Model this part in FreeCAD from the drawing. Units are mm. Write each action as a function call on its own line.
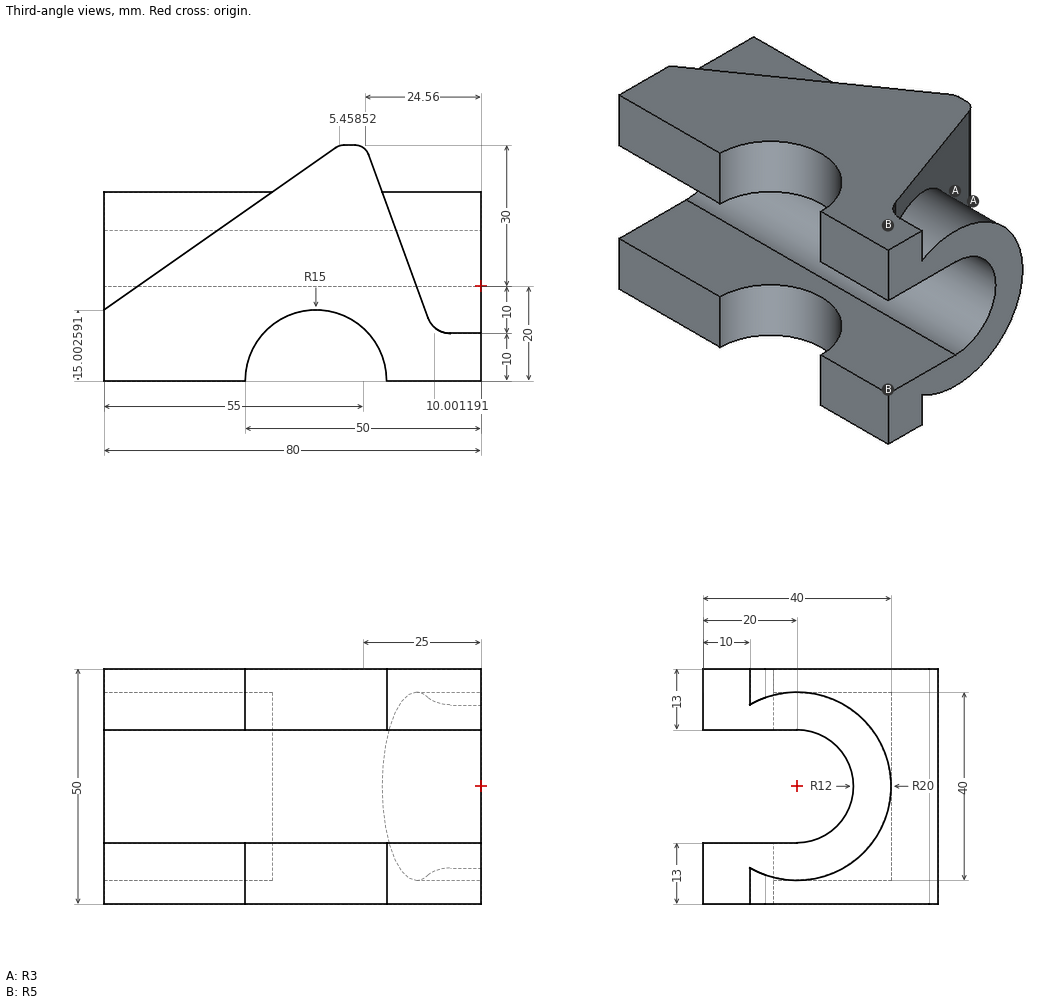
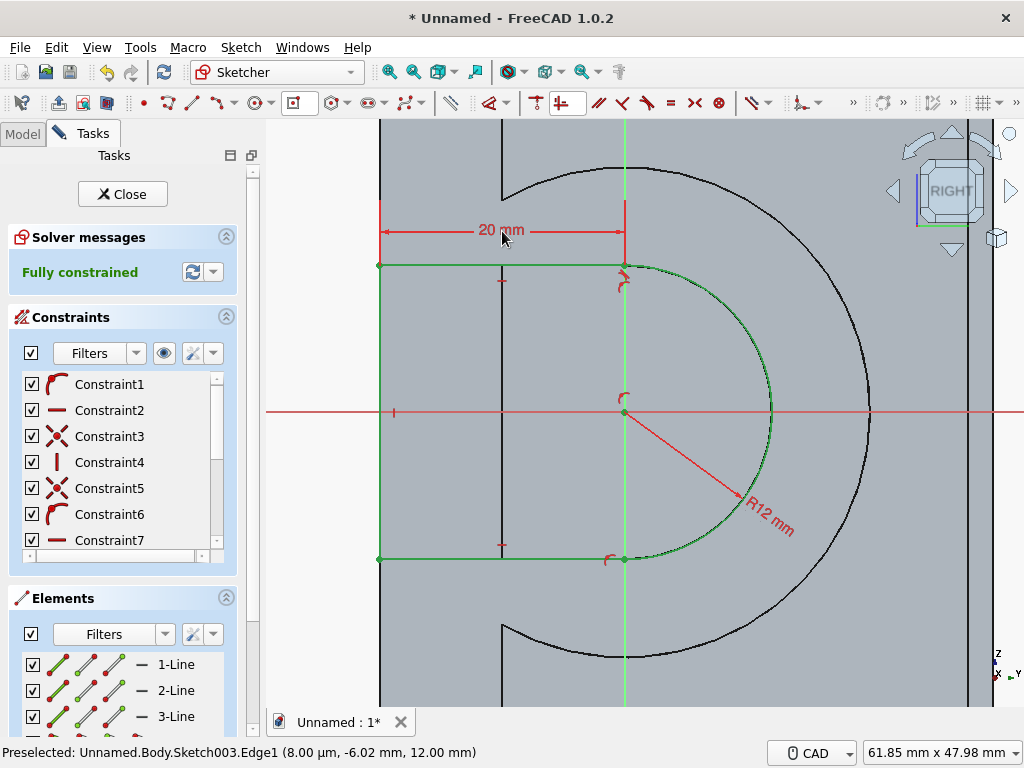
click(123, 194)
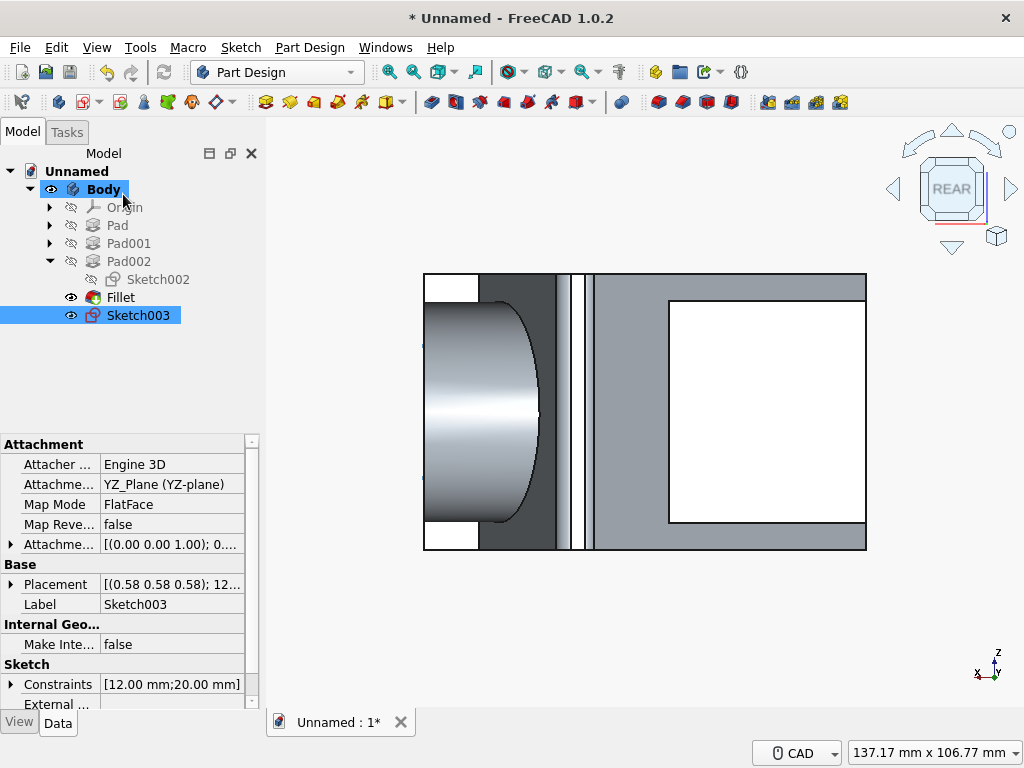
click(432, 102)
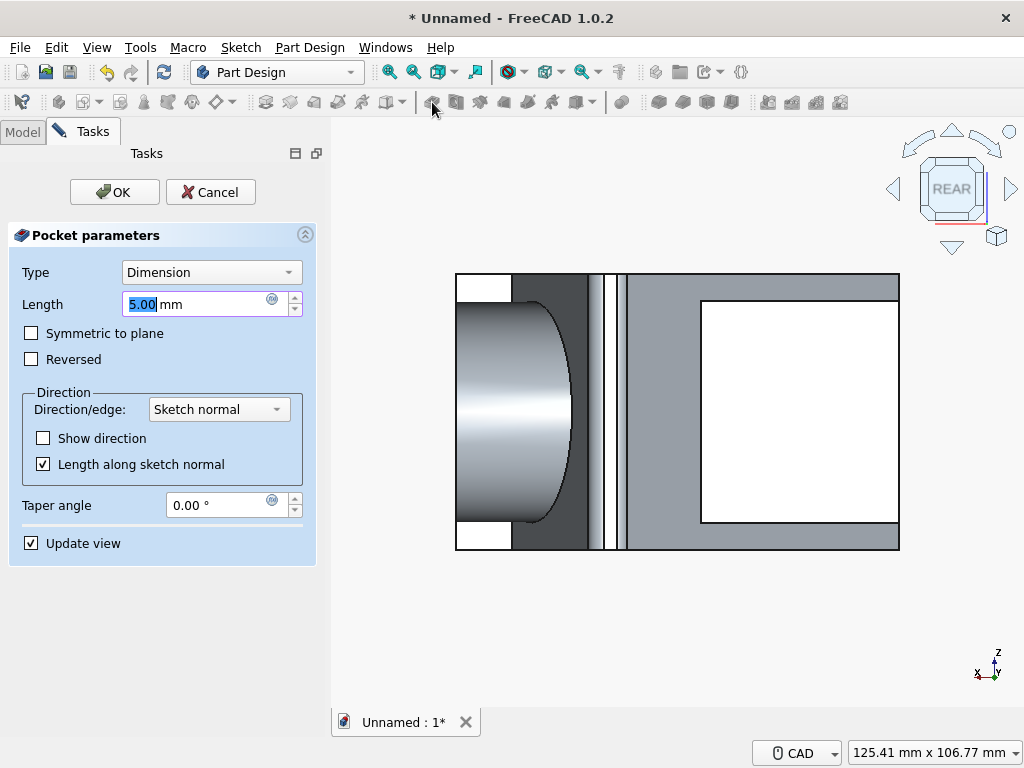
click(212, 272)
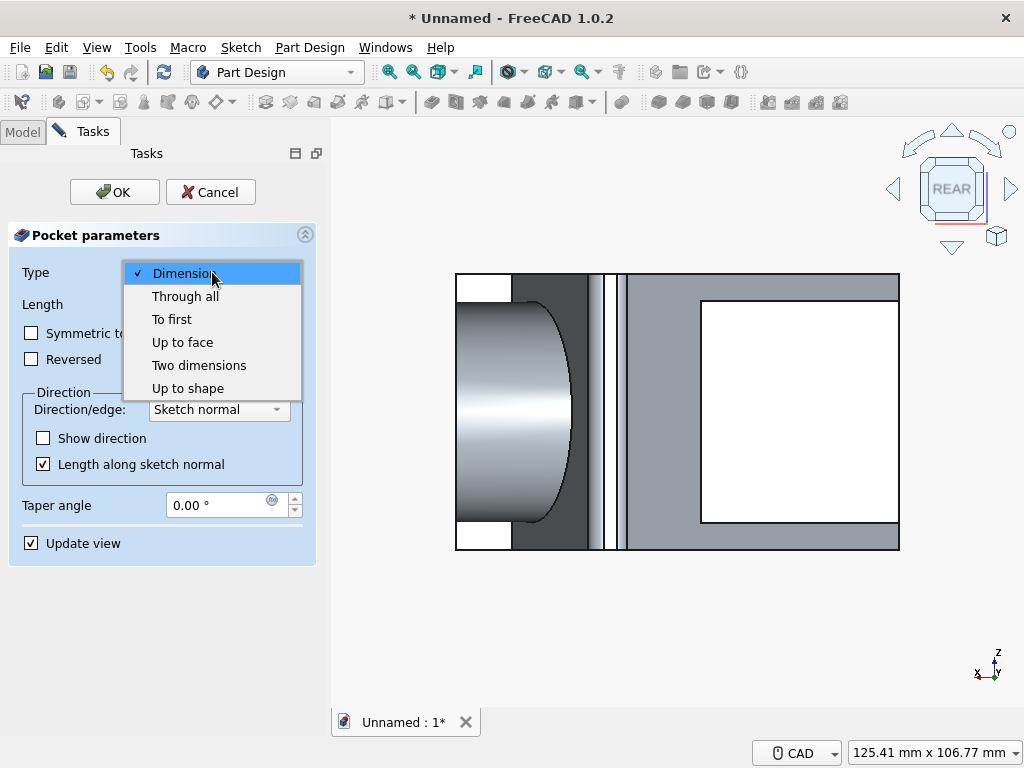
click(212, 296)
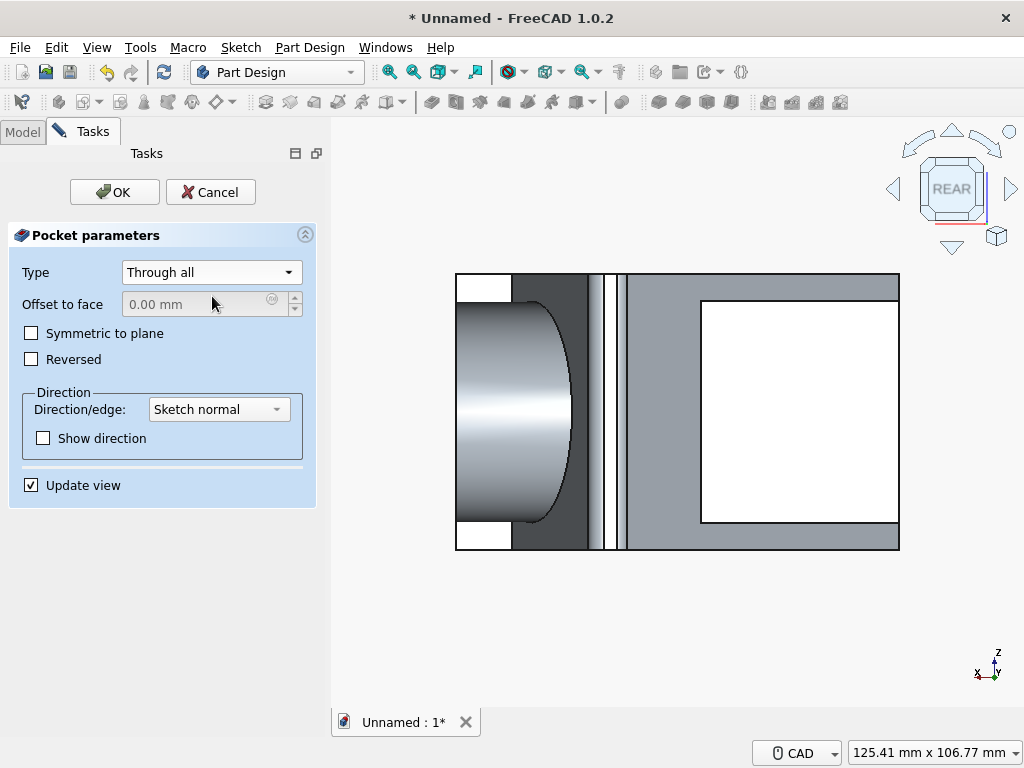
click(115, 192)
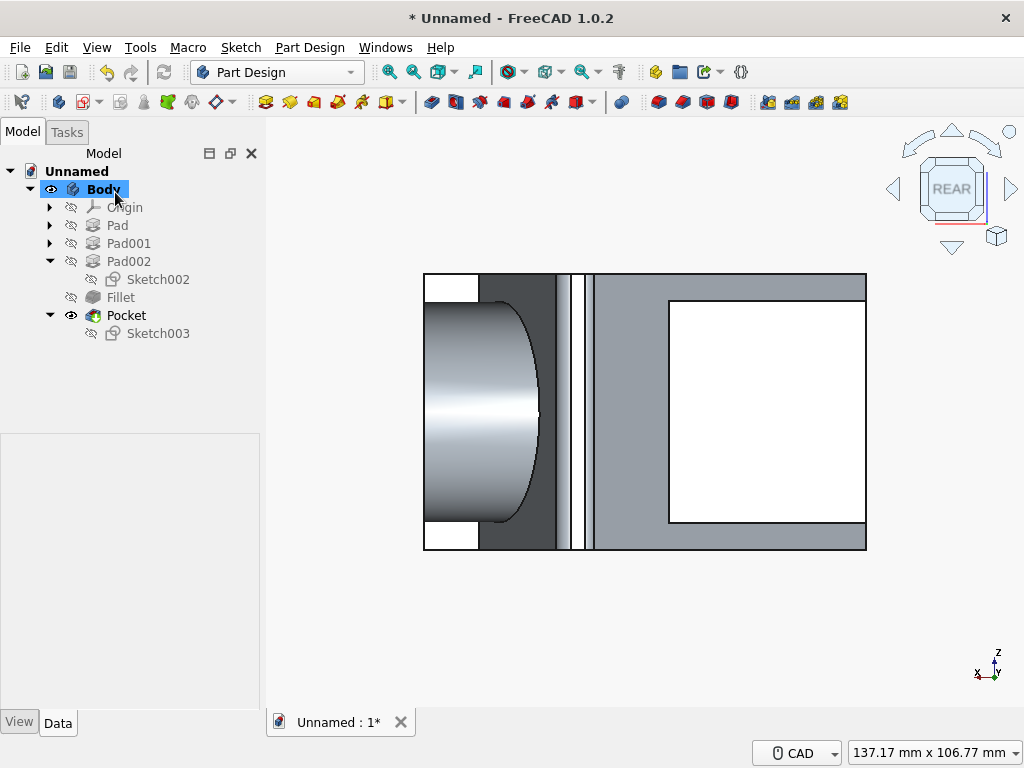
key(0)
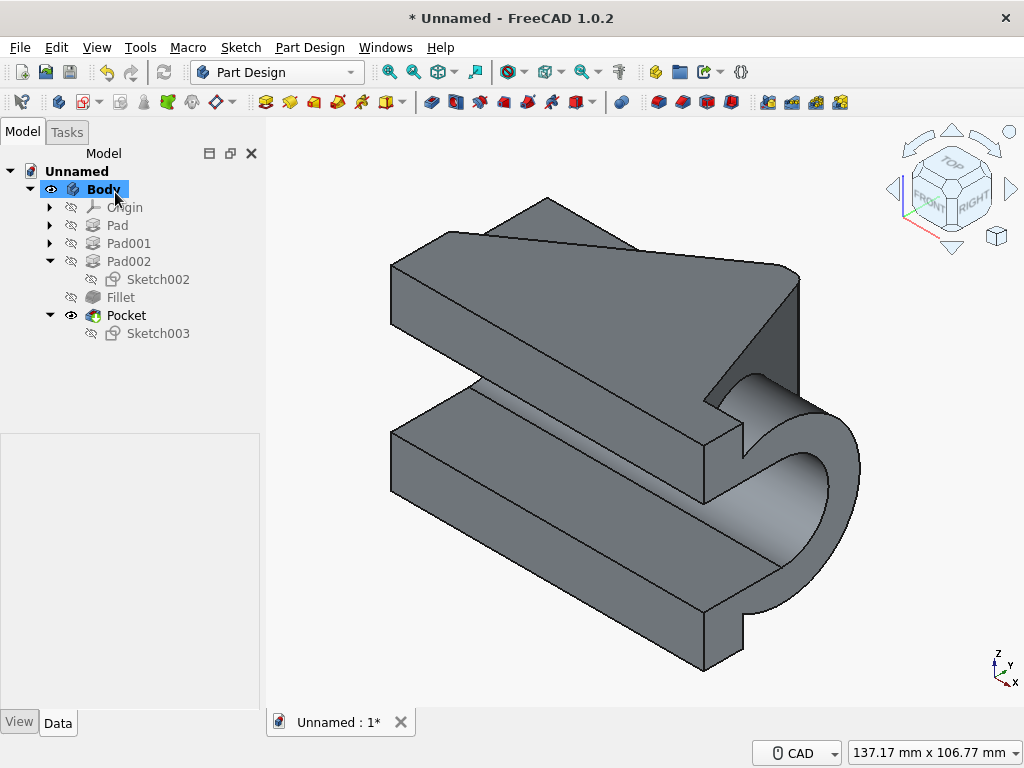
click(617, 314)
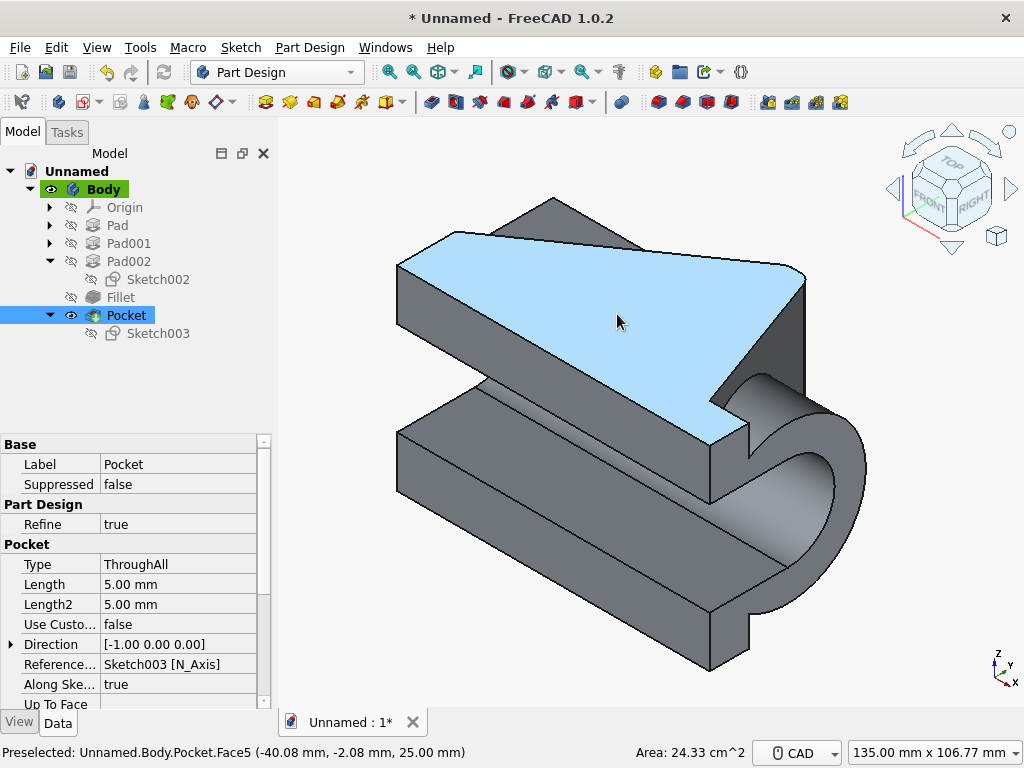
click(84, 102)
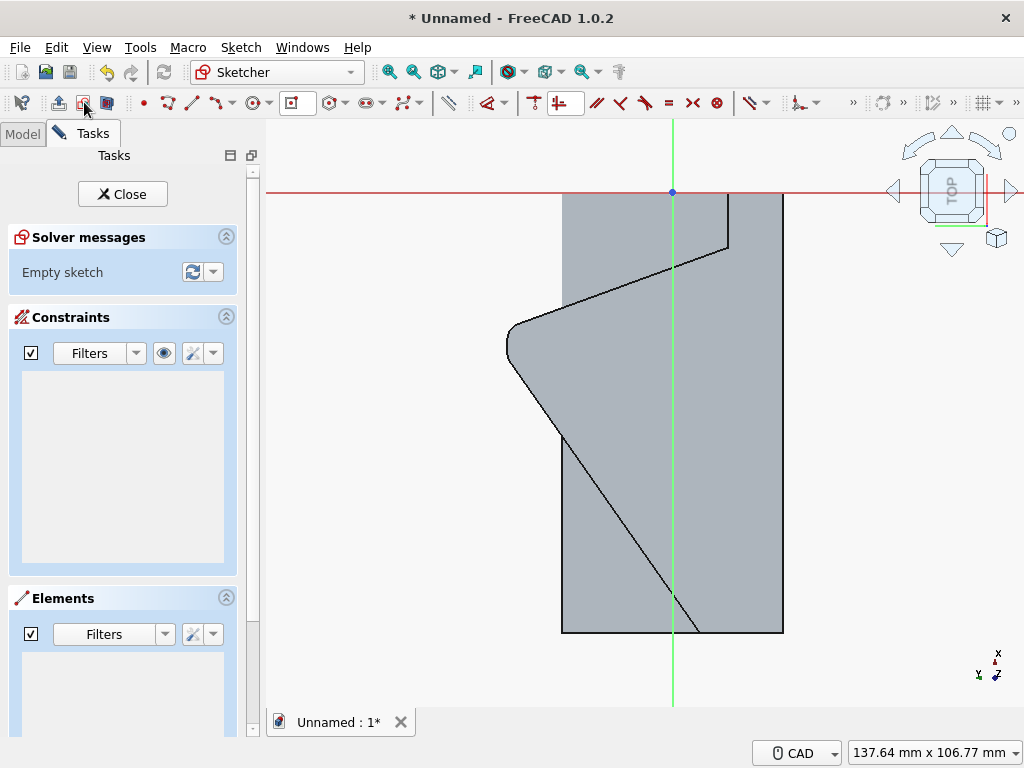
scroll(859, 162, up, 2)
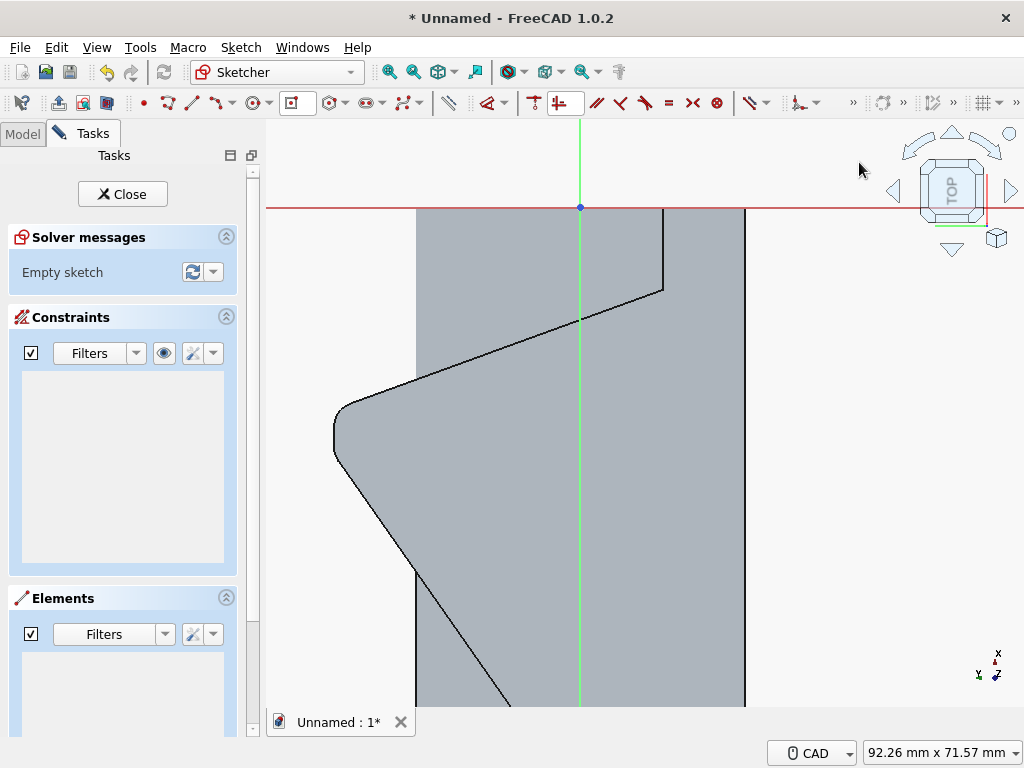
click(192, 104)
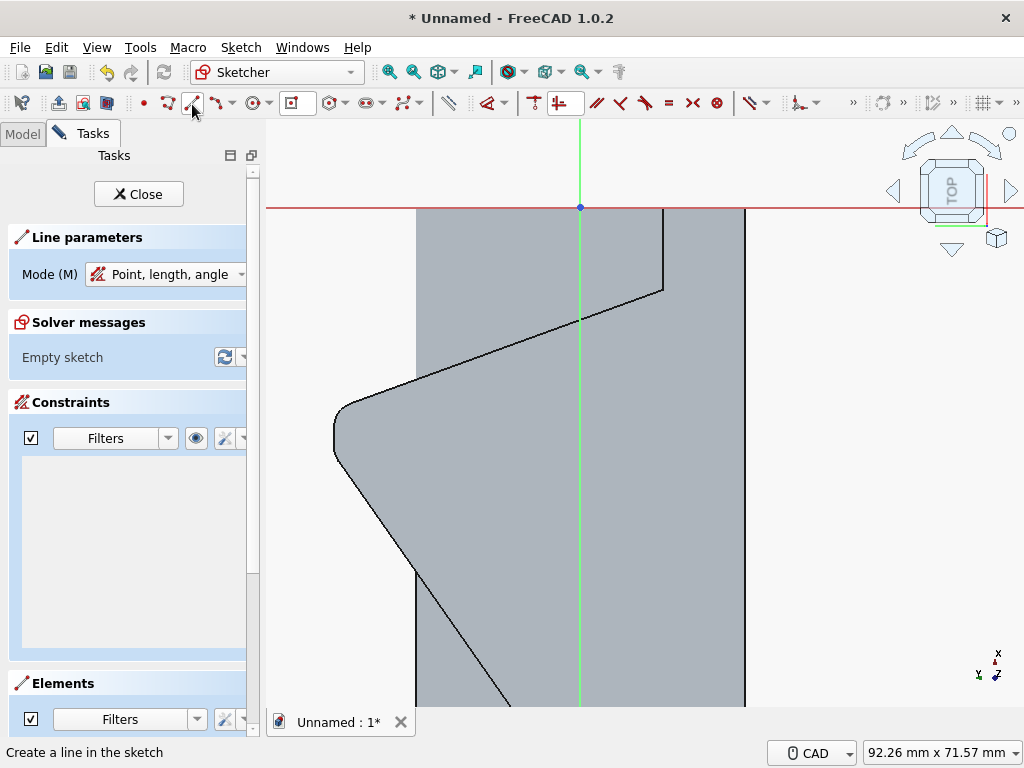
click(745, 619)
click(745, 372)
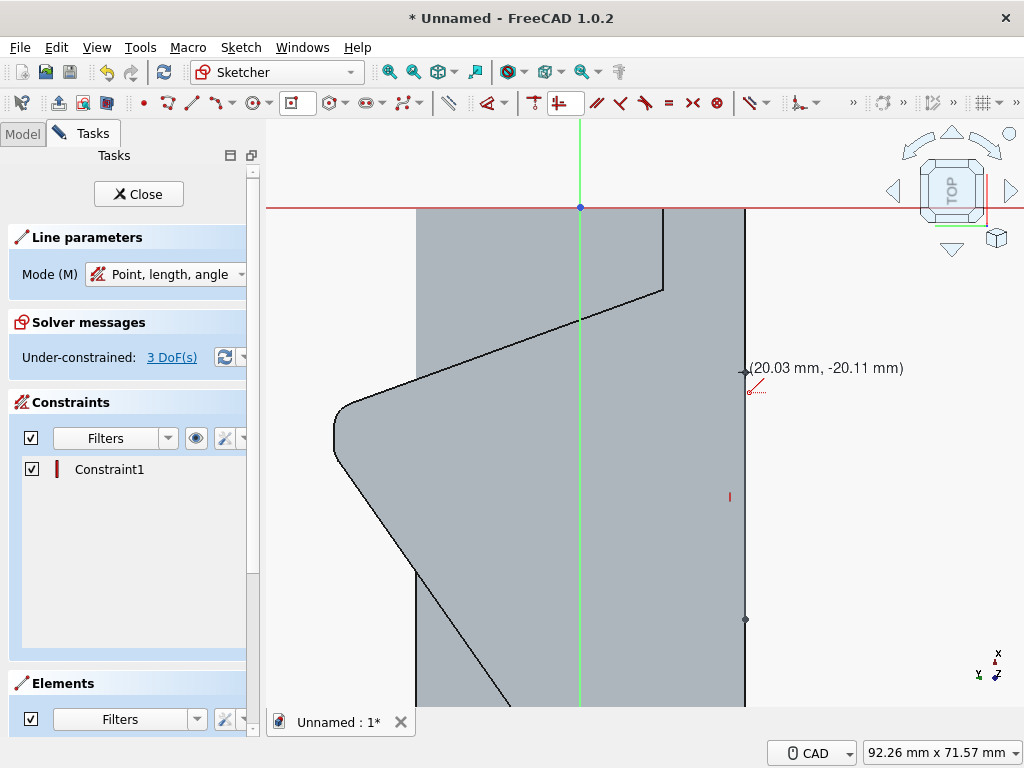
key(g)
key(3)
key(a)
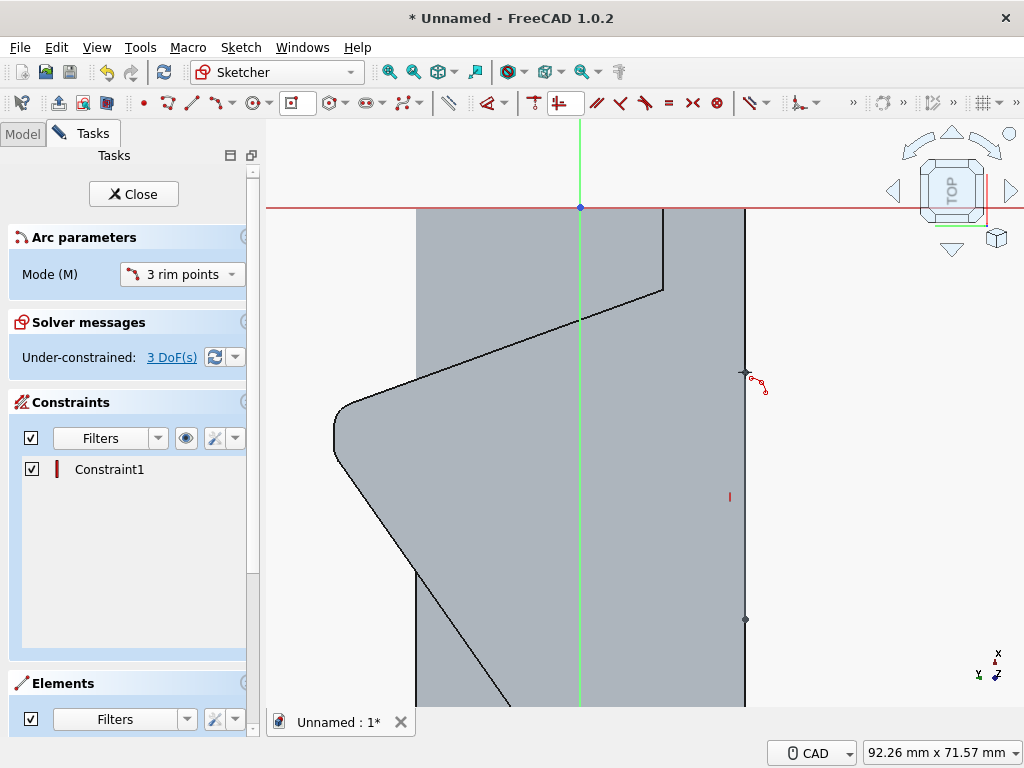
click(745, 373)
click(745, 620)
click(622, 495)
key(Escape)